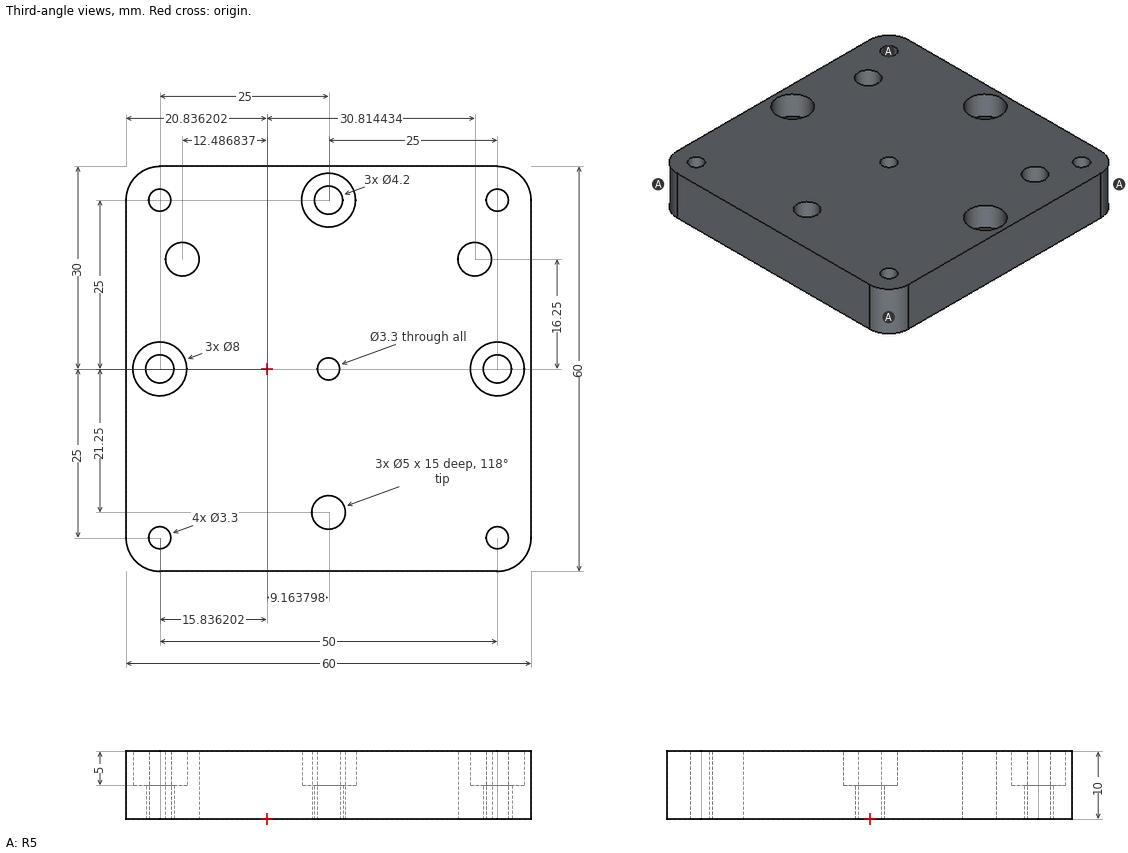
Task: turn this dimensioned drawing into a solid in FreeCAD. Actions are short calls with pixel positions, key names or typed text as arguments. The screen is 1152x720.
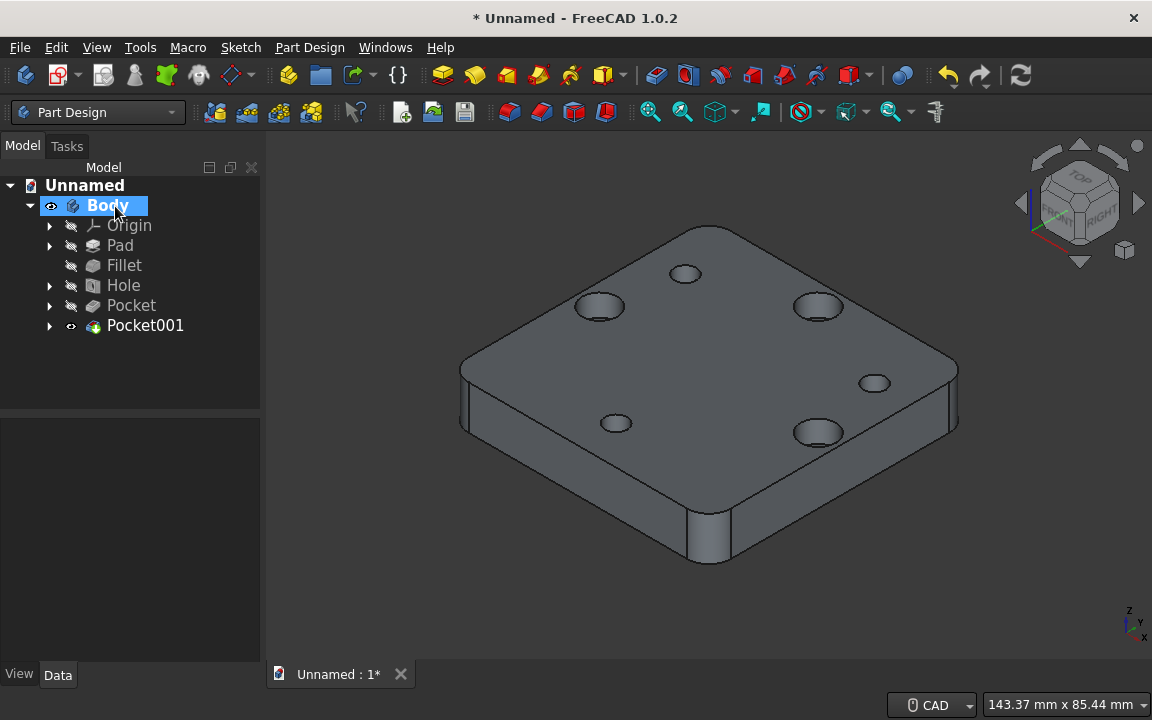
click(709, 369)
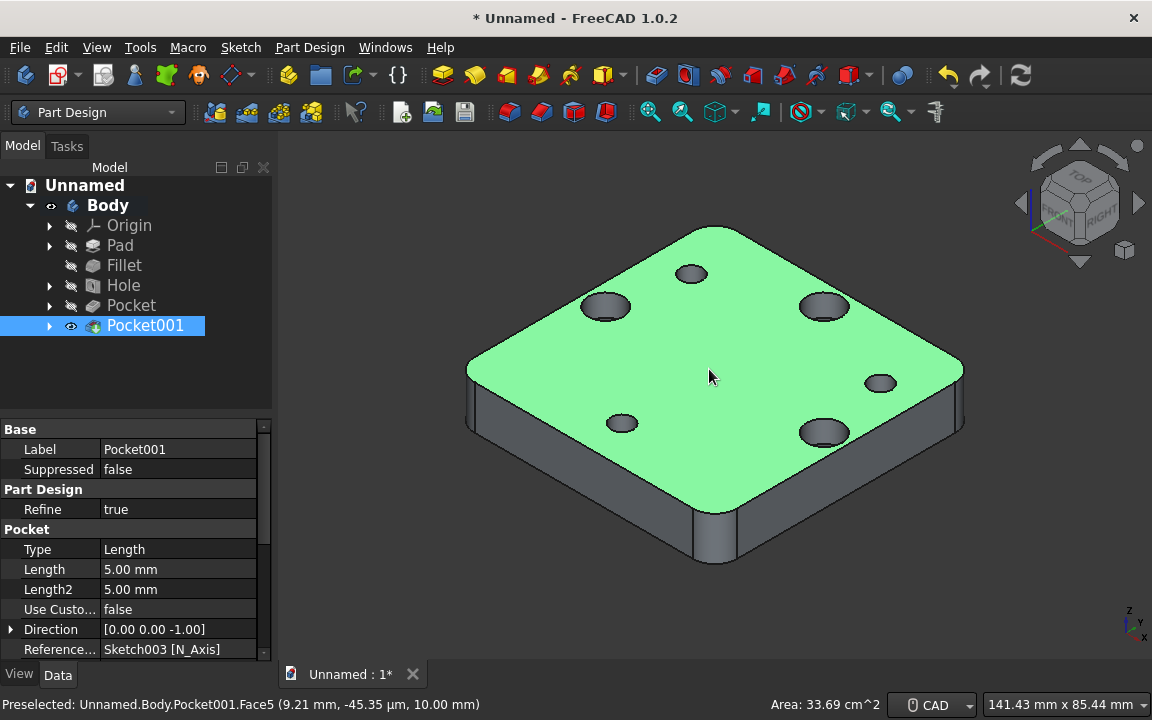
click(58, 76)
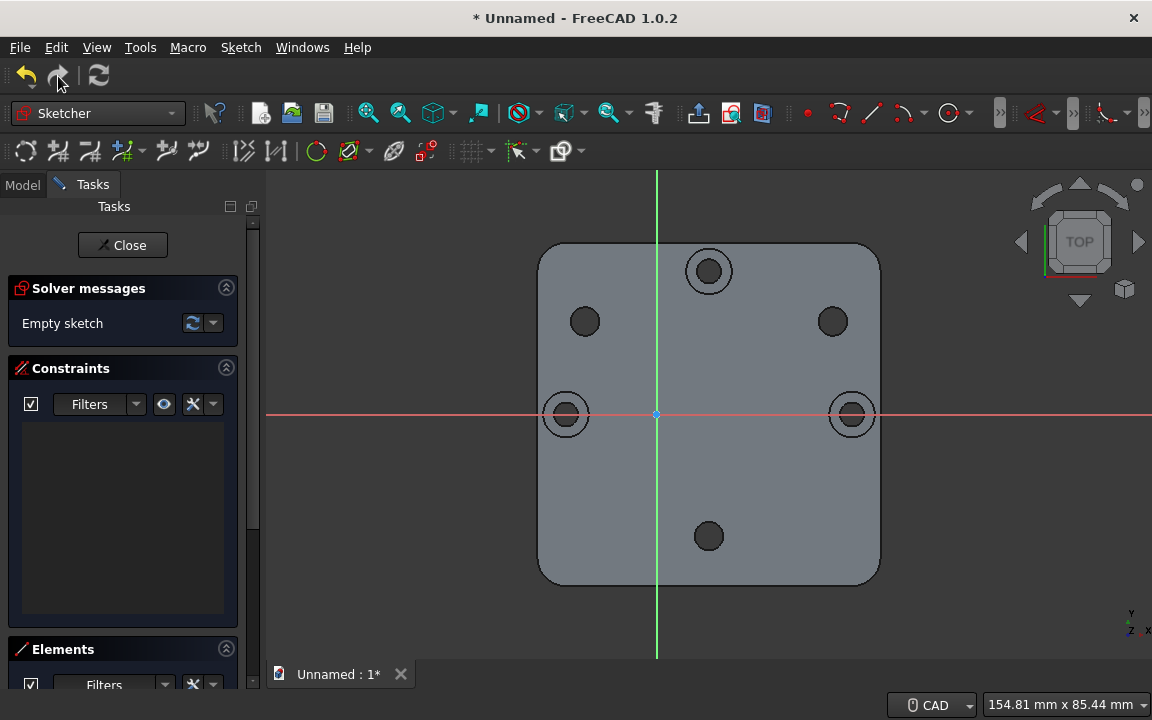
click(950, 114)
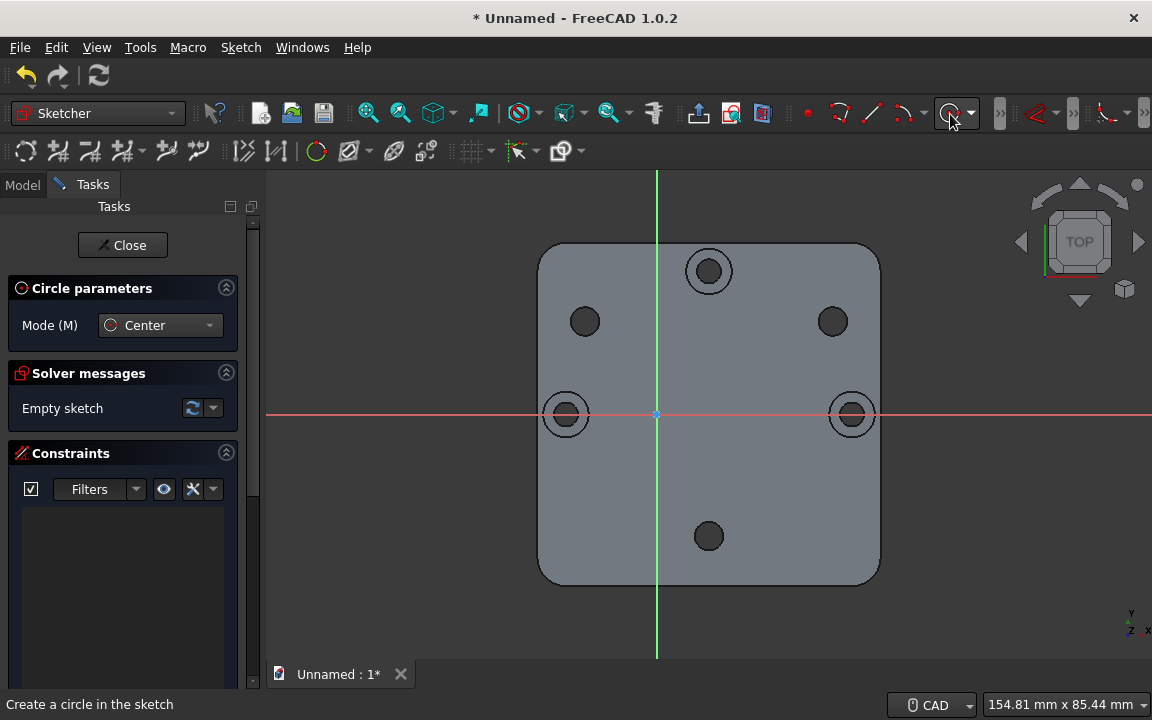
scroll(566, 558, up, 5)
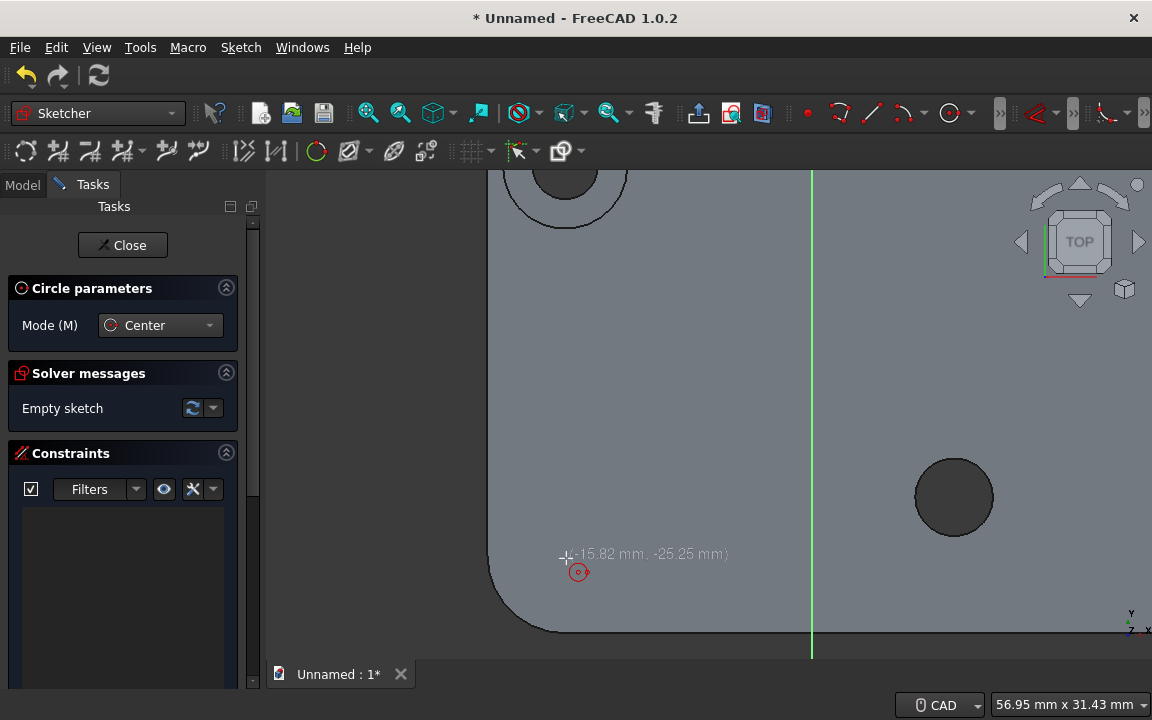
click(565, 555)
move(583, 537)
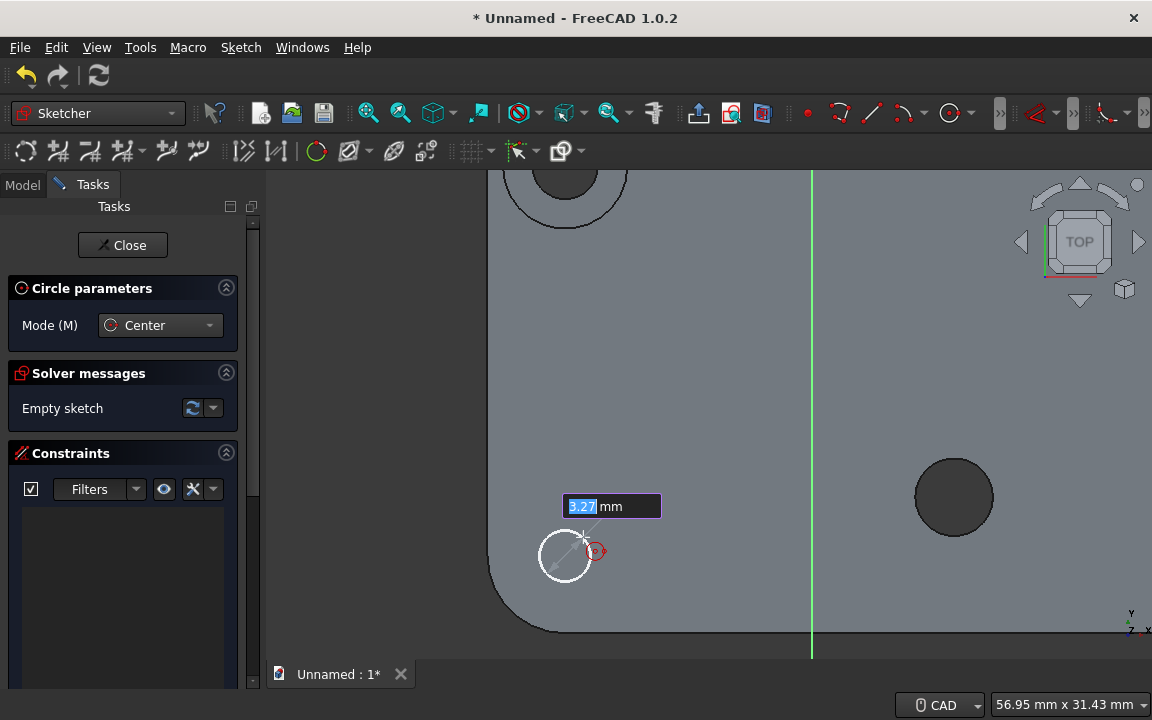
text(3.3)
key(Return)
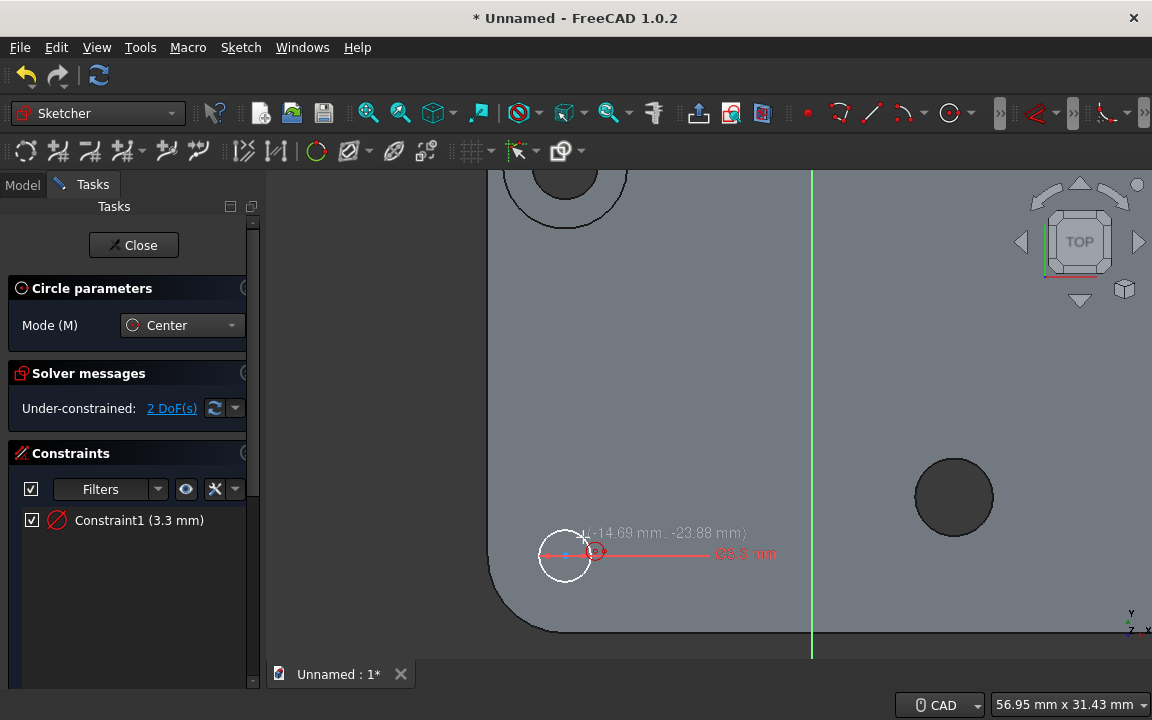
scroll(458, 559, down, 5)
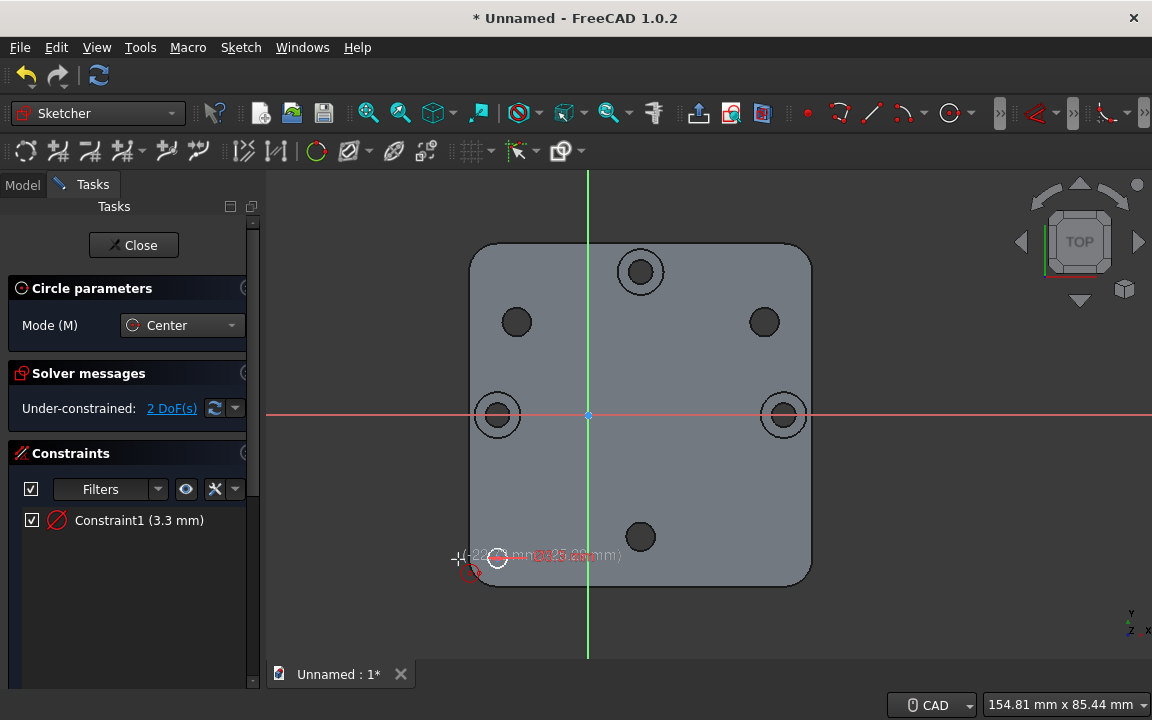
scroll(784, 558, up, 5)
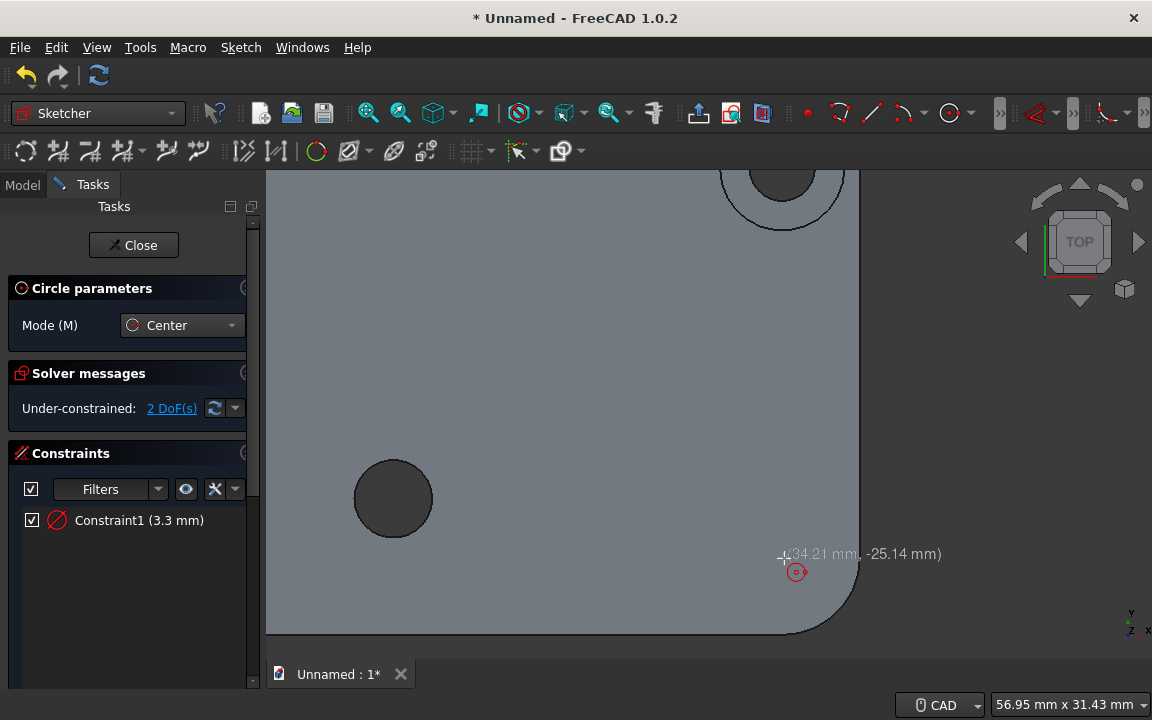
click(782, 557)
move(800, 539)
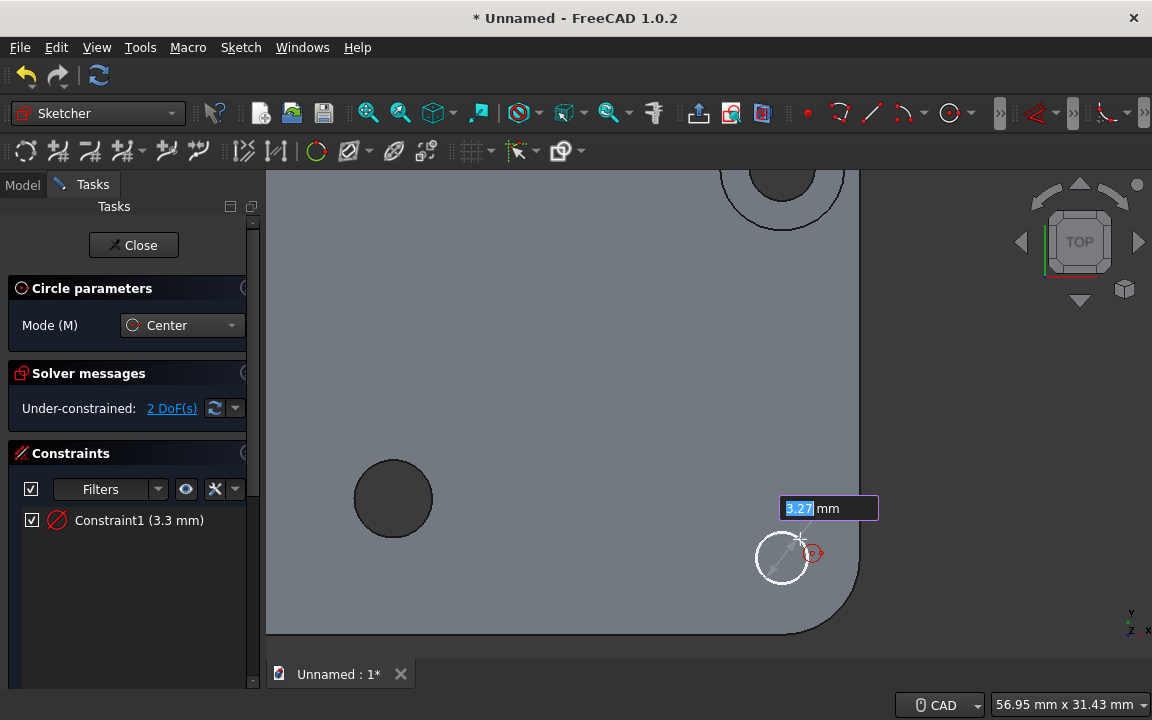
text(3.3)
key(Return)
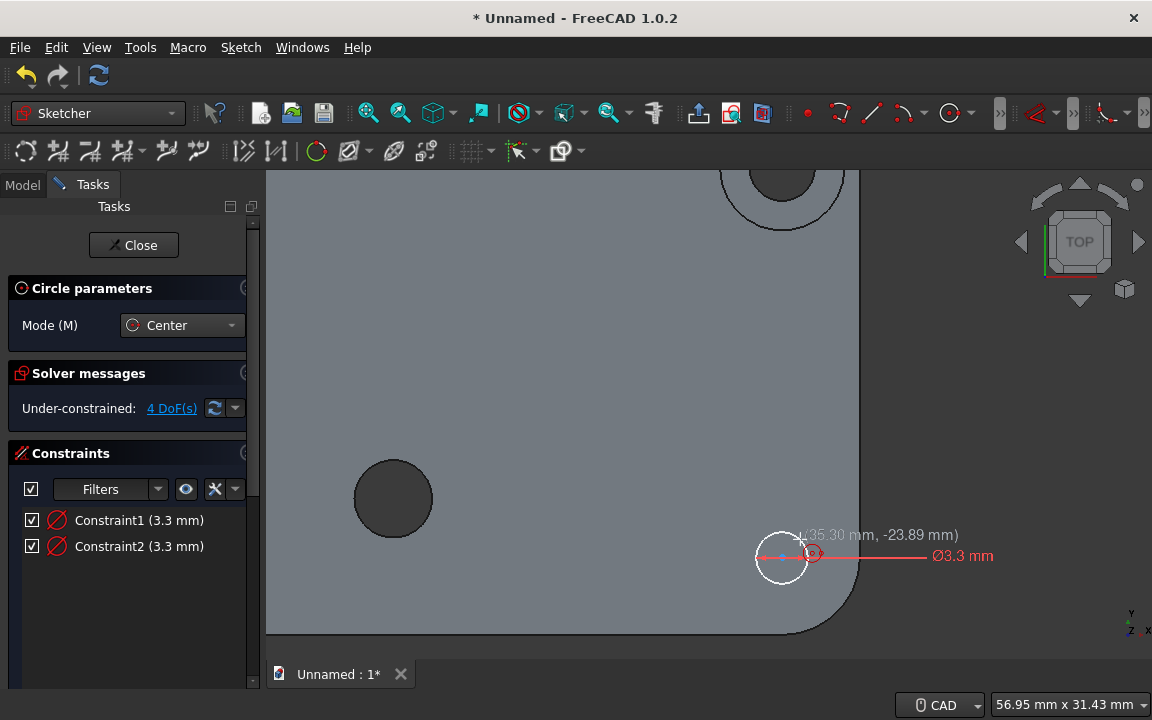
scroll(784, 558, down, 5)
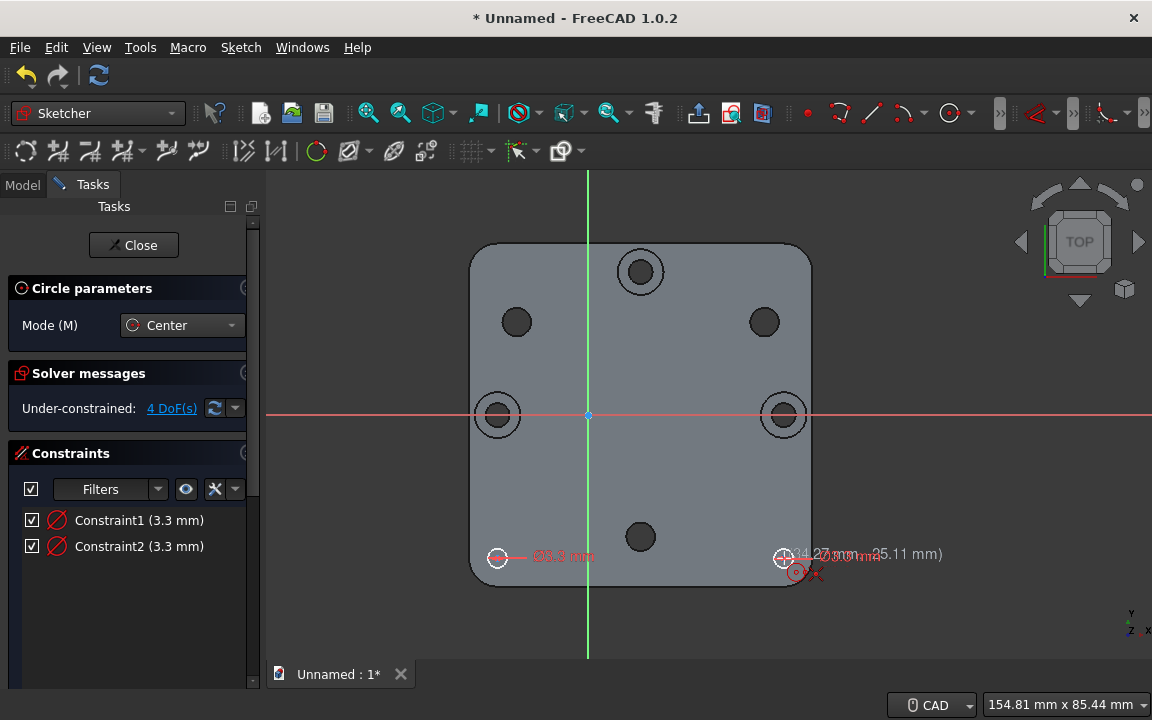
scroll(784, 272, up, 5)